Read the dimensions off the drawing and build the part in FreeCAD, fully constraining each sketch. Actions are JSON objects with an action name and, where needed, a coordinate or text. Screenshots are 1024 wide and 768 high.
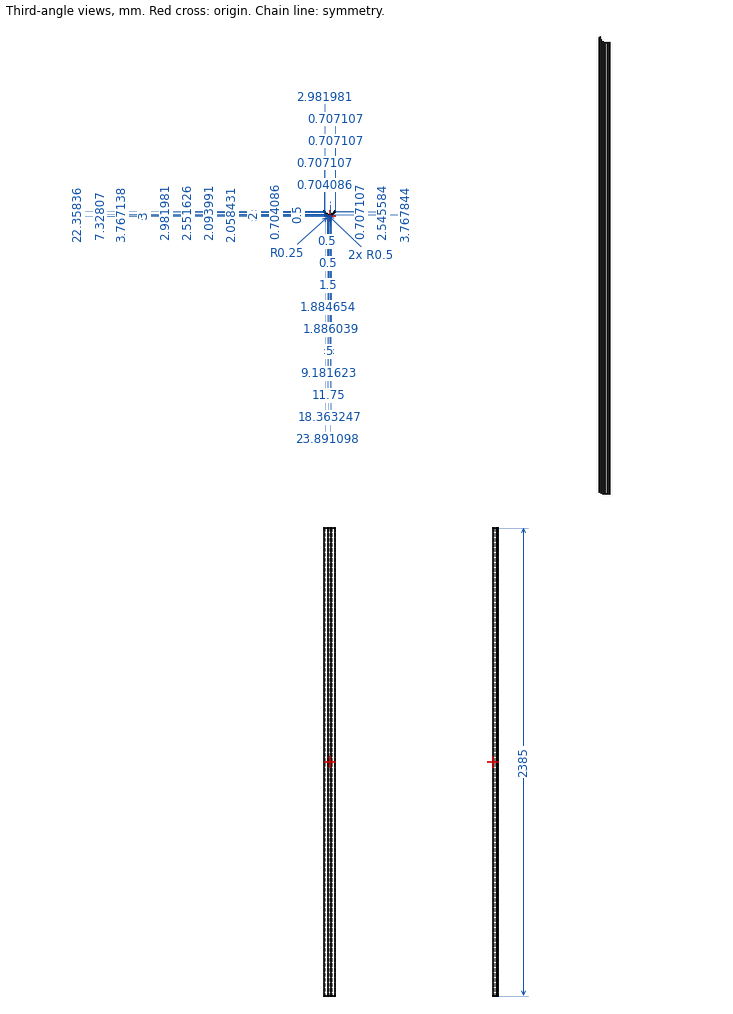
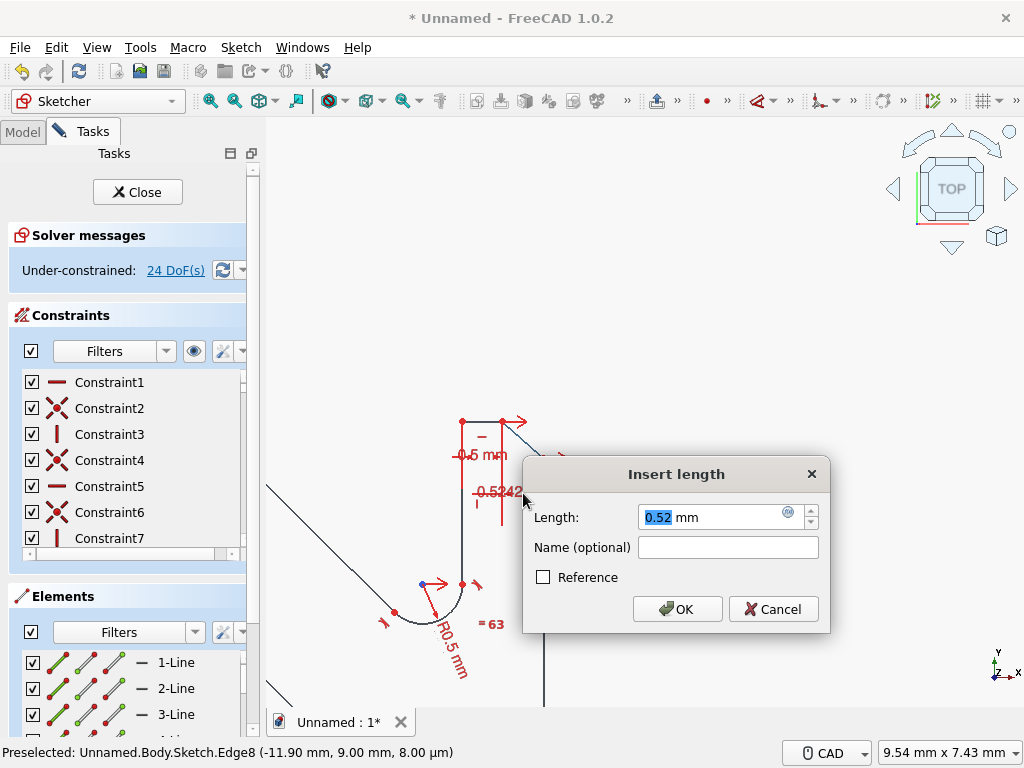
{"action": "type", "text": "0.5"}
{"action": "key", "text": "Return"}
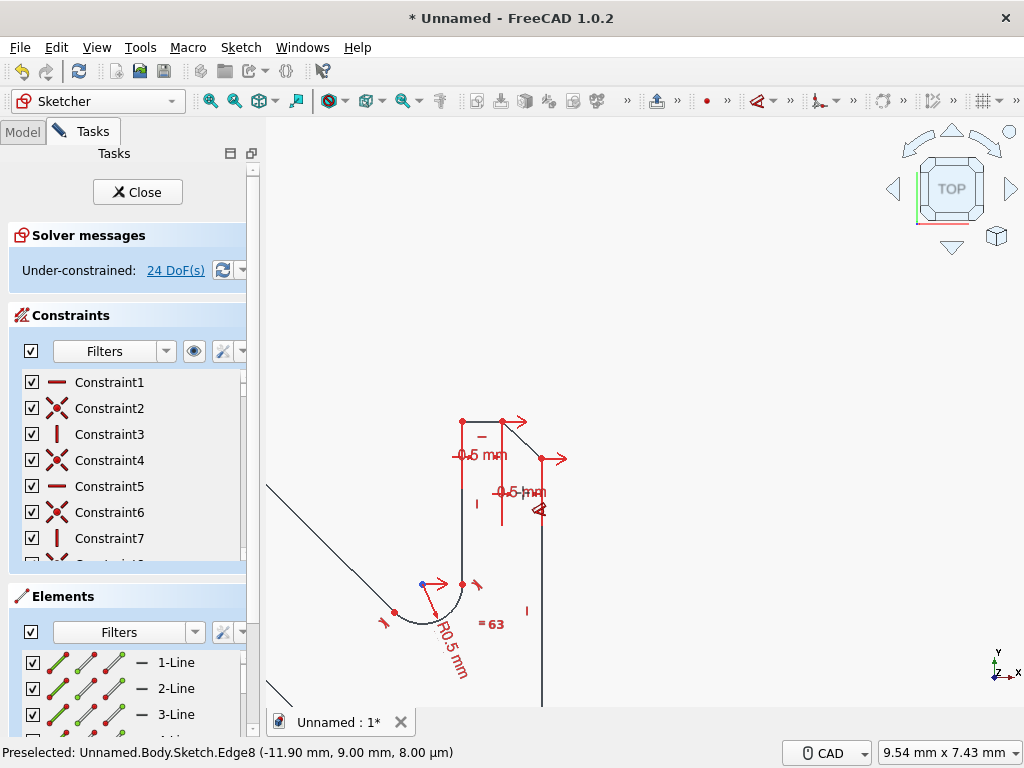
{"action": "left_click", "coordinate": [530, 448]}
{"action": "left_click", "coordinate": [576, 440]}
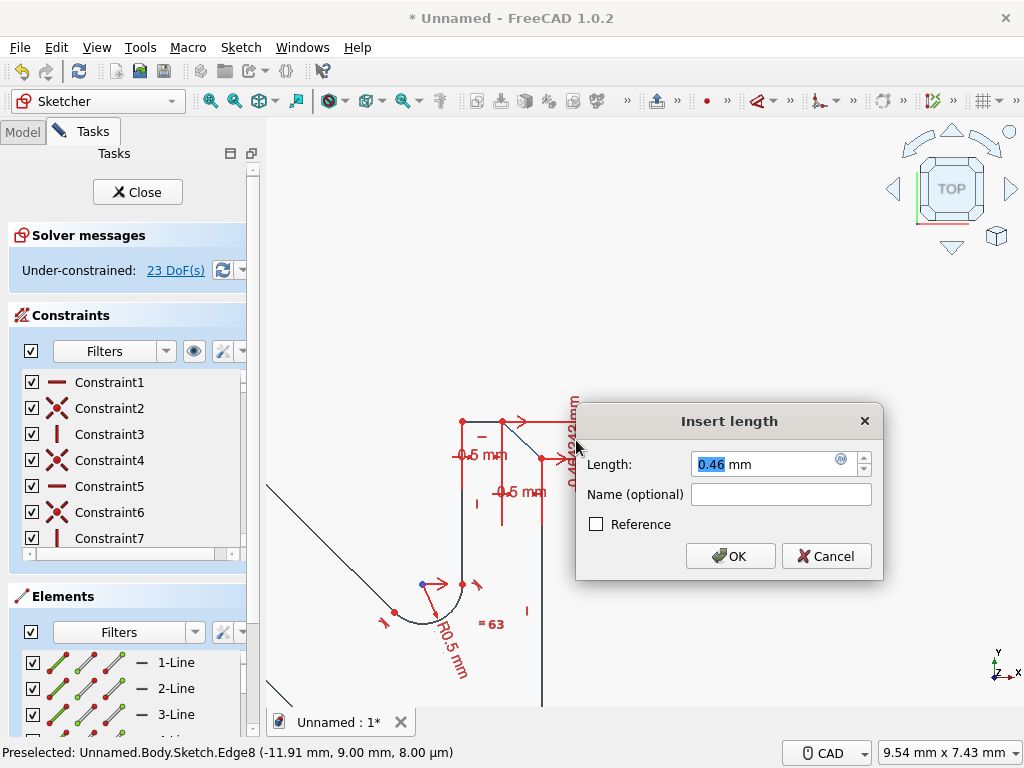
{"action": "type", "text": "0.5"}
{"action": "key", "text": "Return"}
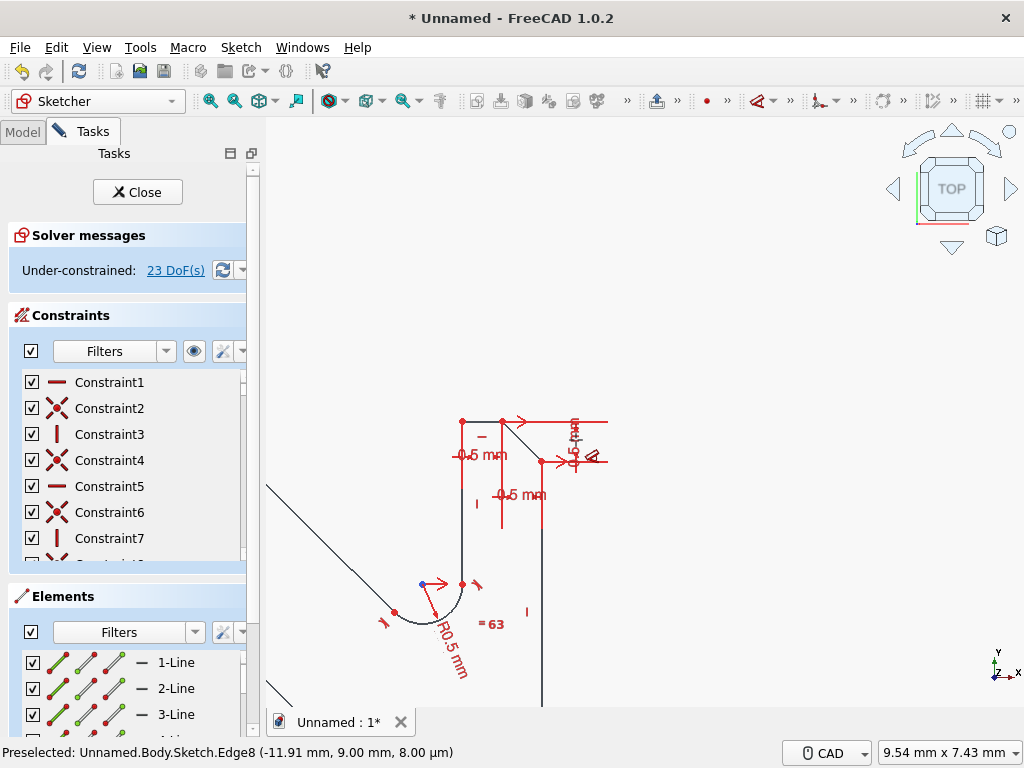
{"action": "scroll", "coordinate": [487, 426], "scroll_direction": "down", "scroll_amount": 12}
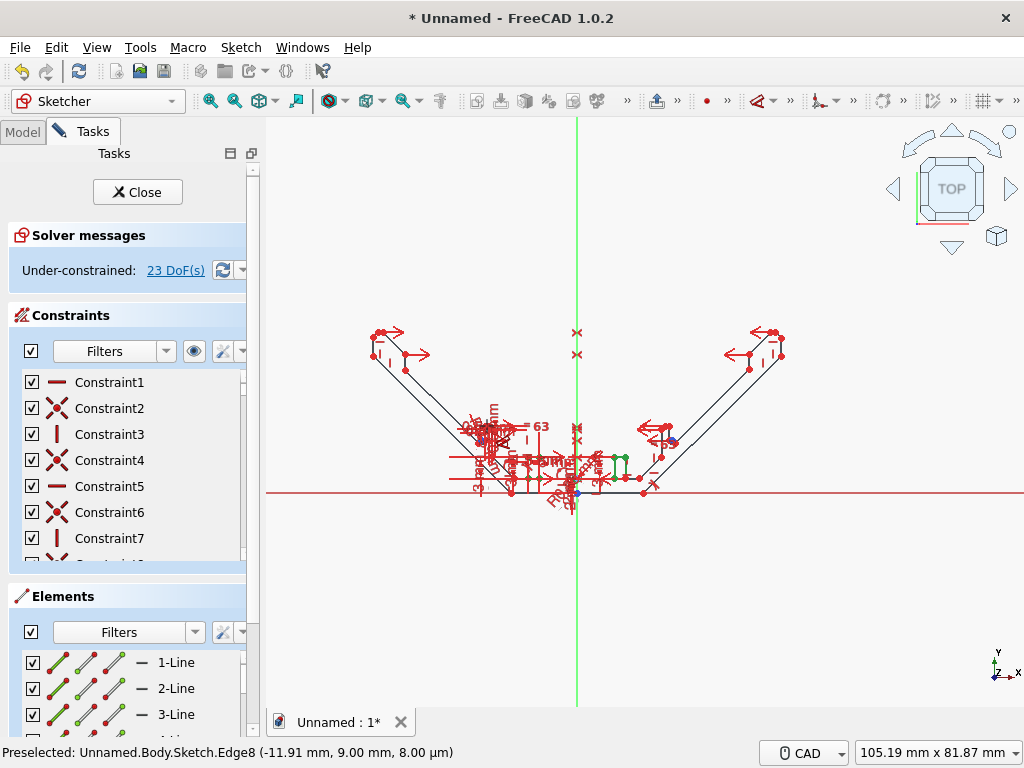
{"action": "left_click", "coordinate": [492, 457]}
{"action": "left_click", "coordinate": [535, 527]}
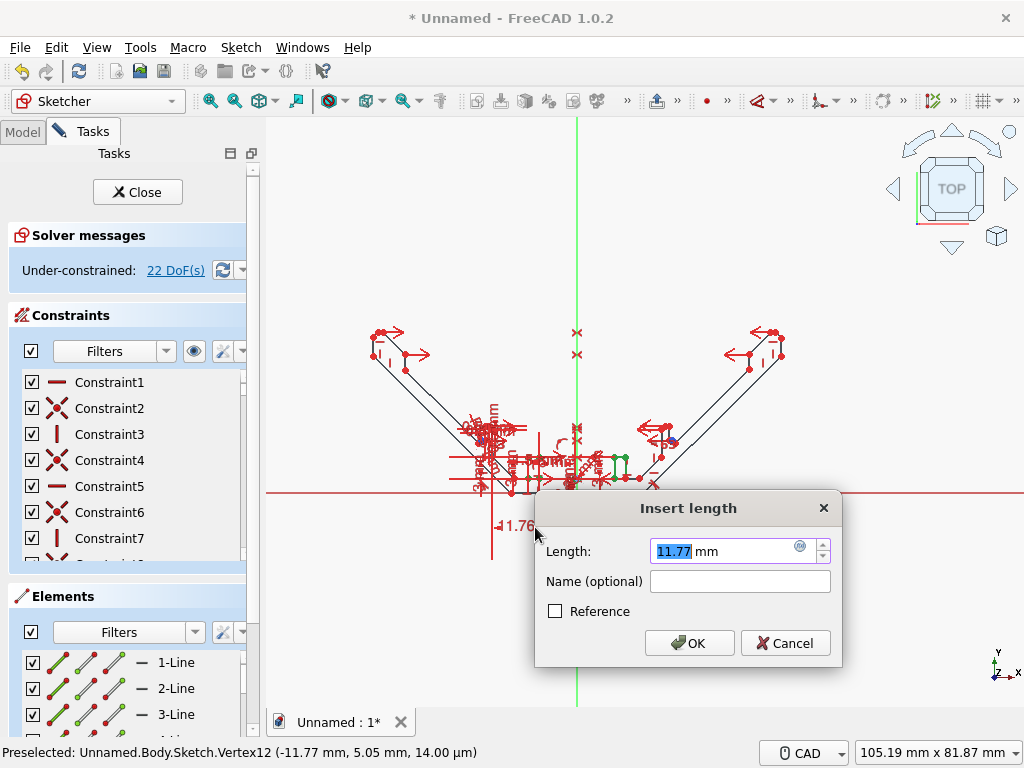
{"action": "type", "text": "11.75"}
{"action": "key", "text": "Return"}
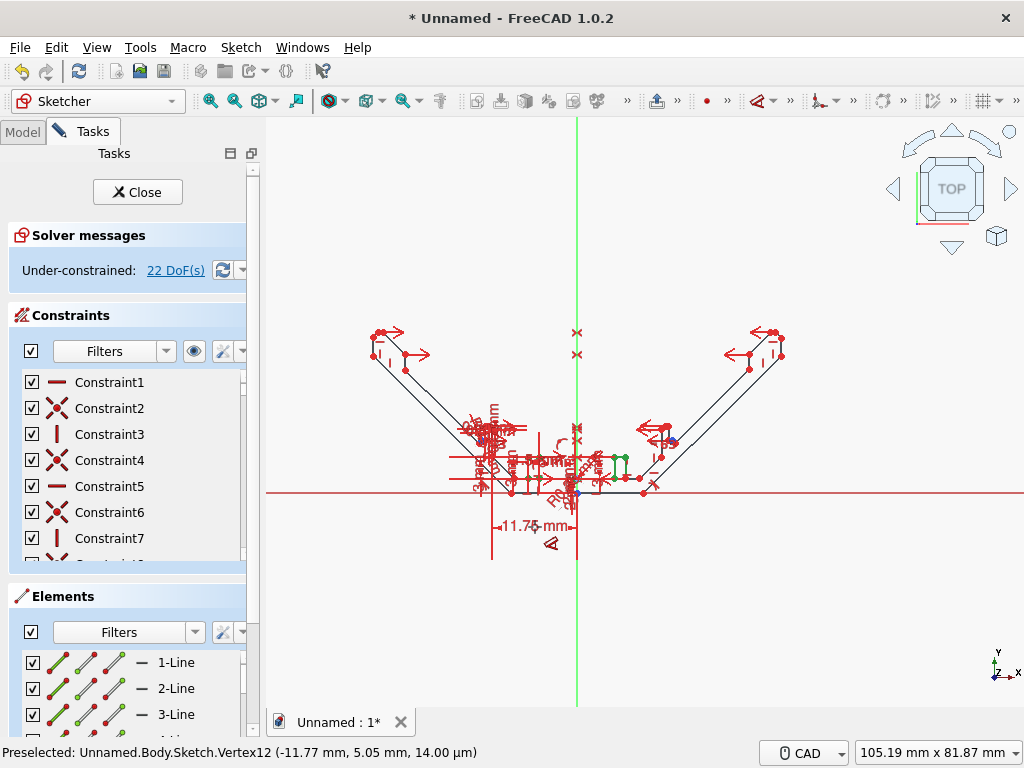
{"action": "scroll", "coordinate": [521, 479], "scroll_direction": "up", "scroll_amount": 6}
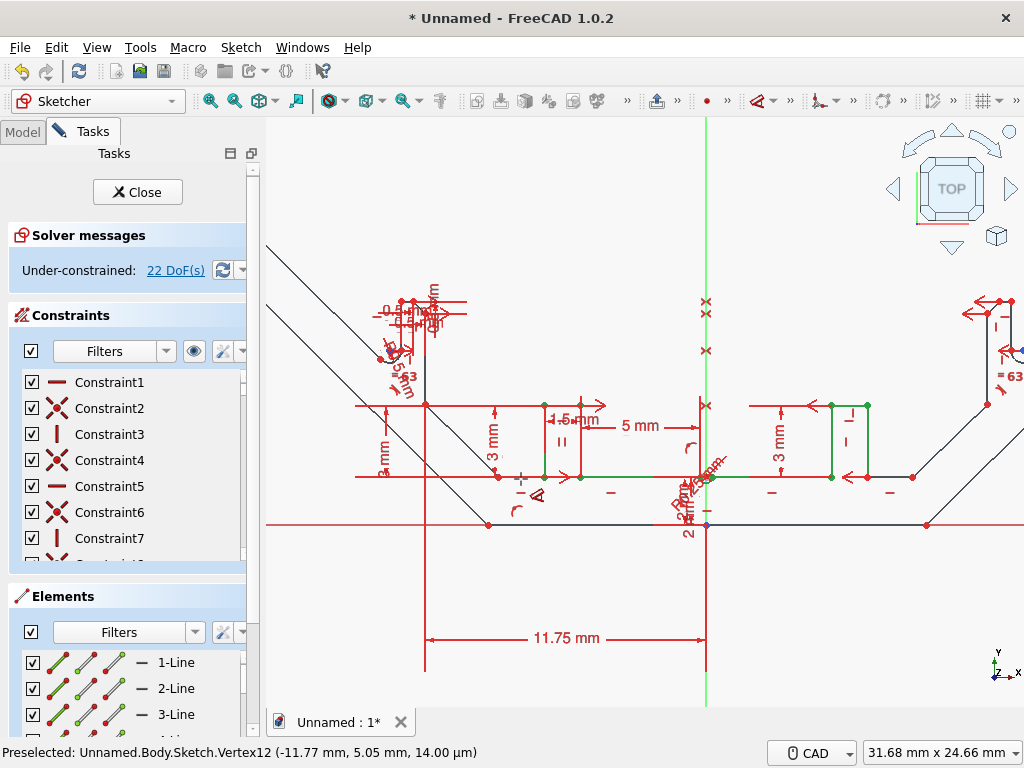
{"action": "left_click", "coordinate": [522, 477]}
{"action": "left_click", "coordinate": [522, 511]}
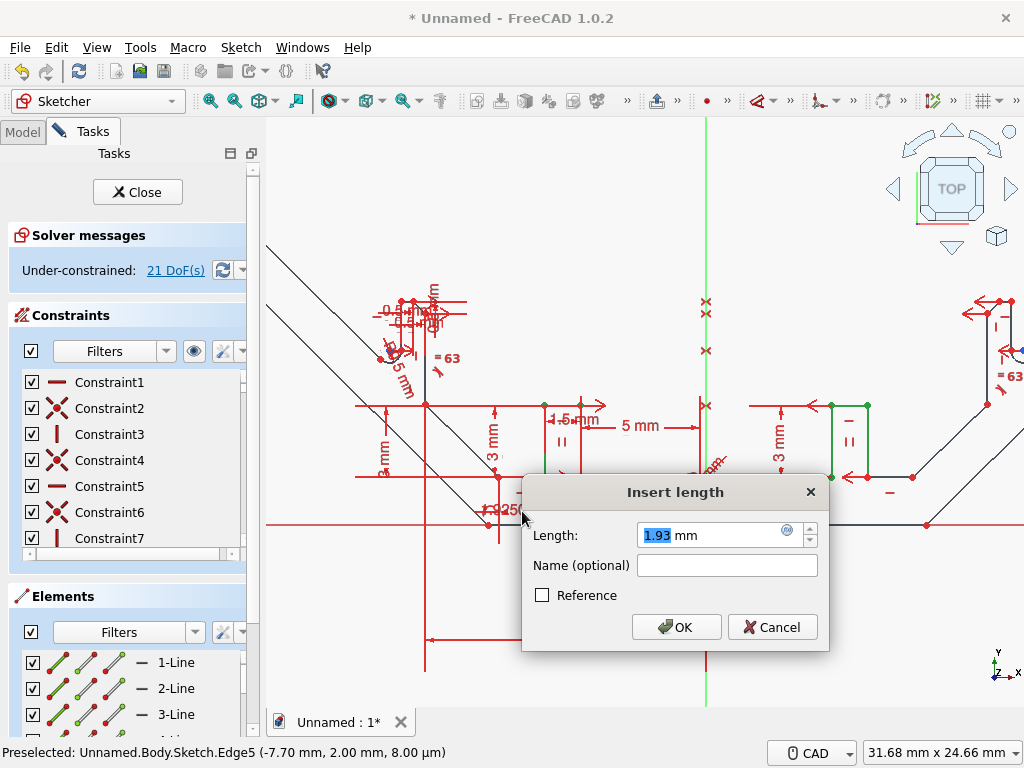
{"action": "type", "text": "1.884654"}
{"action": "key", "text": "Return"}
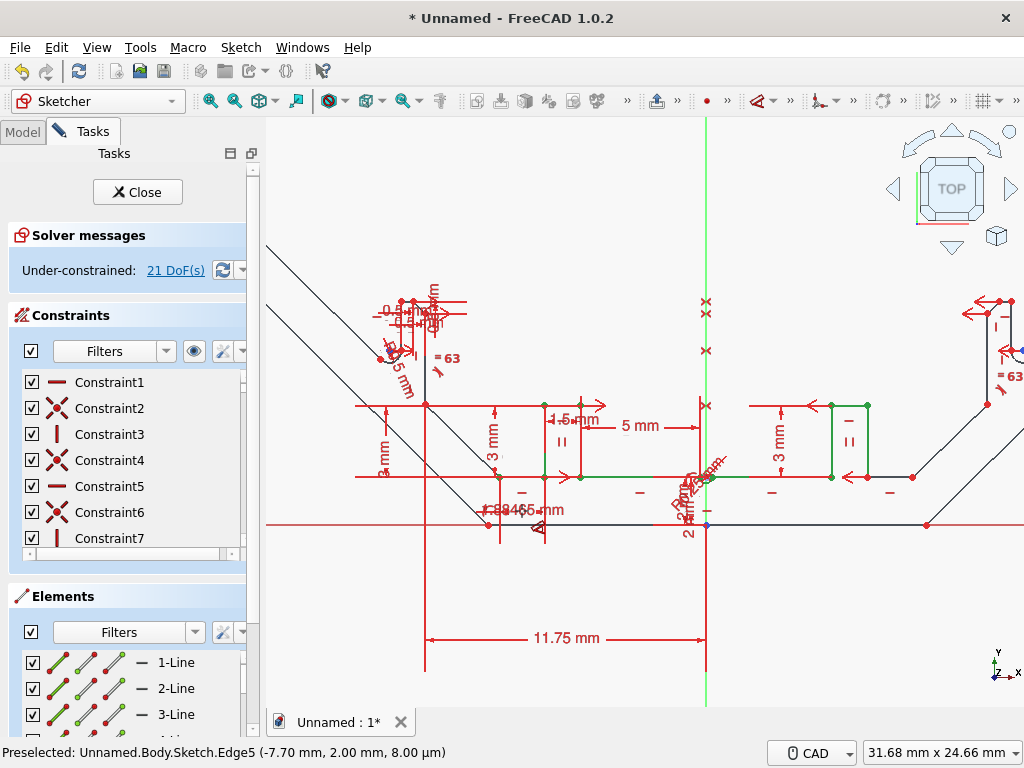
{"action": "left_click", "coordinate": [425, 377]}
{"action": "left_click", "coordinate": [483, 359]}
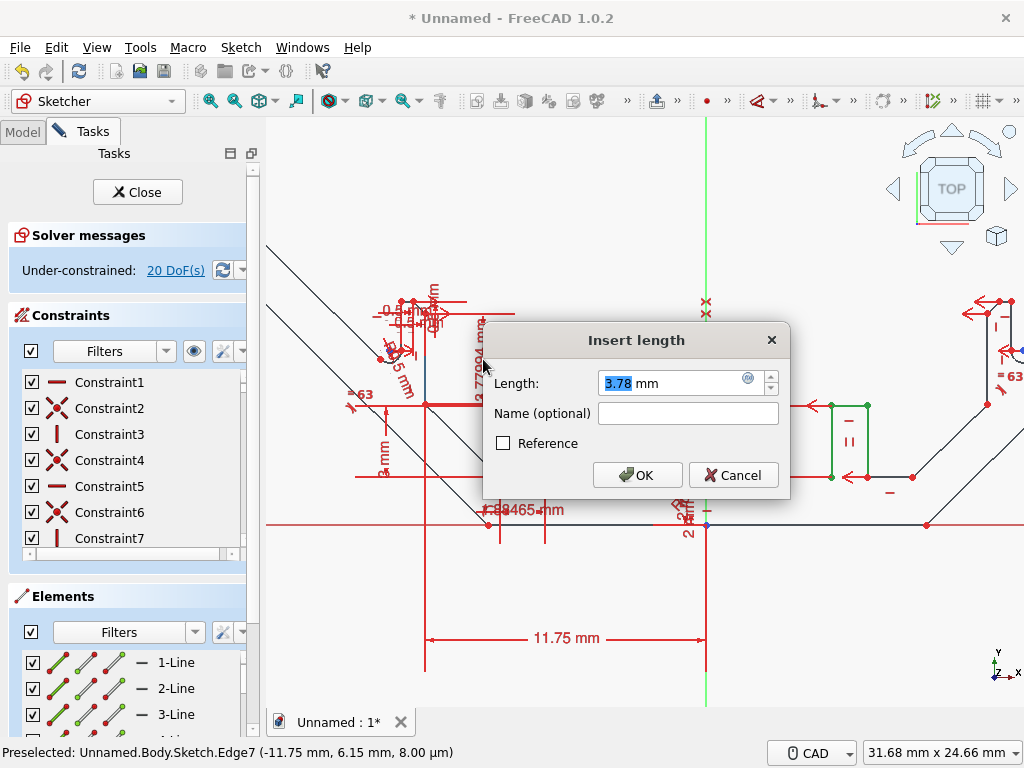
{"action": "type", "text": "3.767138"}
{"action": "key", "text": "Return"}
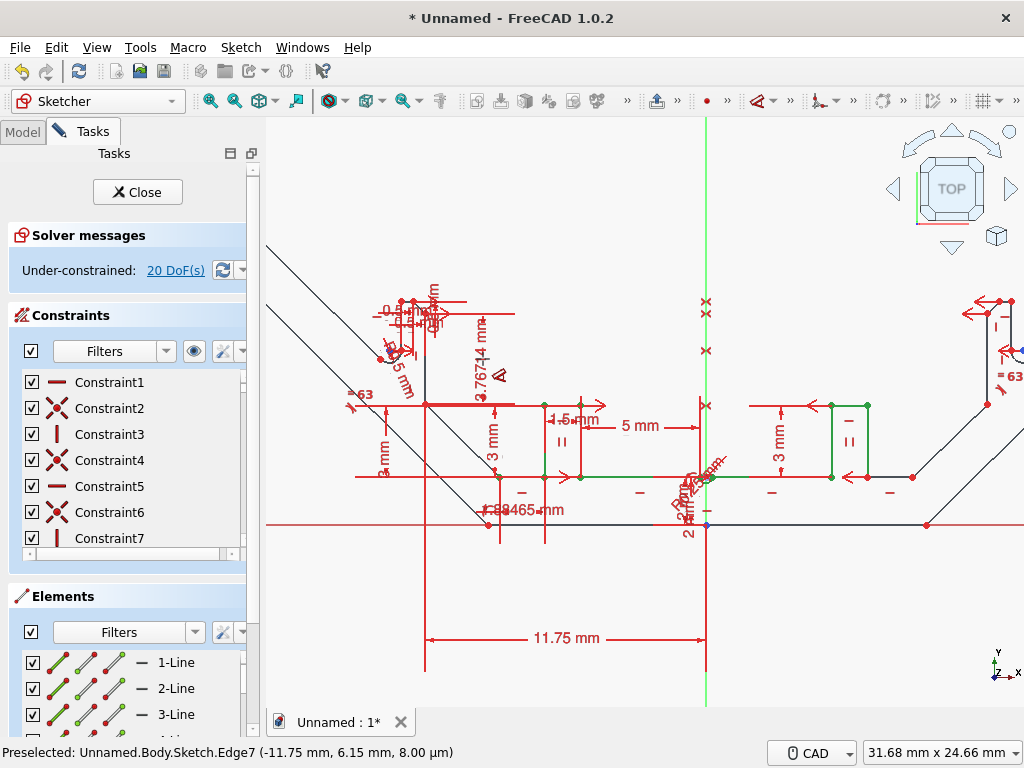
{"action": "left_click", "coordinate": [401, 317]}
{"action": "left_click", "coordinate": [343, 343]}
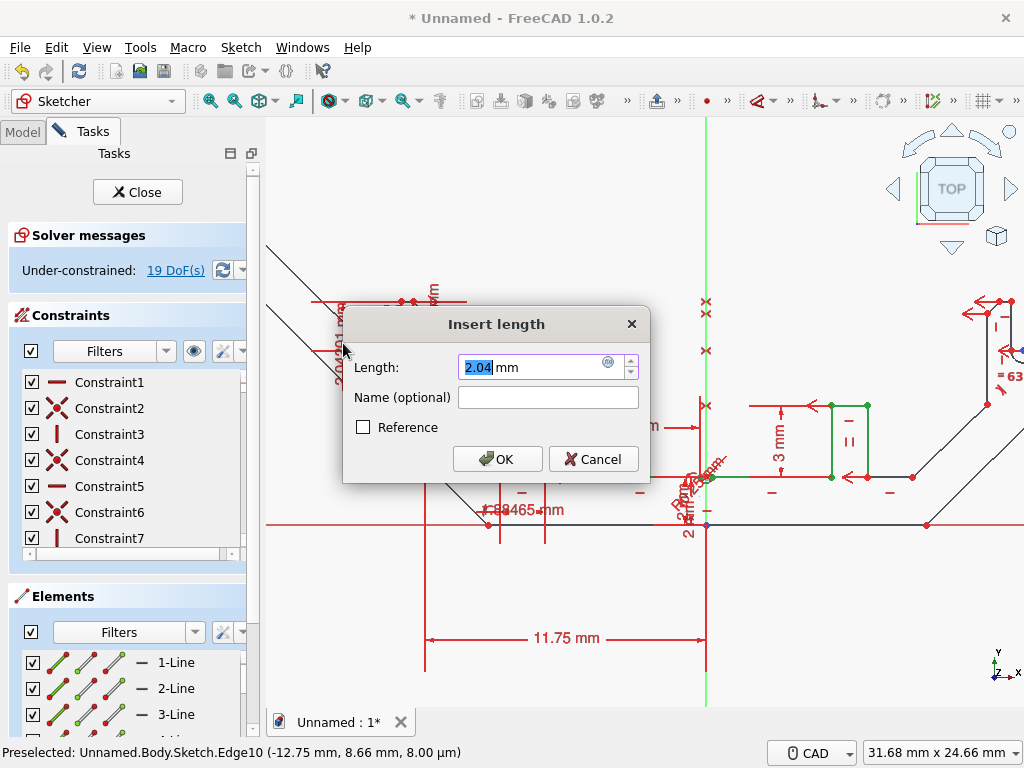
{"action": "type", "text": "2.058431"}
{"action": "key", "text": "Return"}